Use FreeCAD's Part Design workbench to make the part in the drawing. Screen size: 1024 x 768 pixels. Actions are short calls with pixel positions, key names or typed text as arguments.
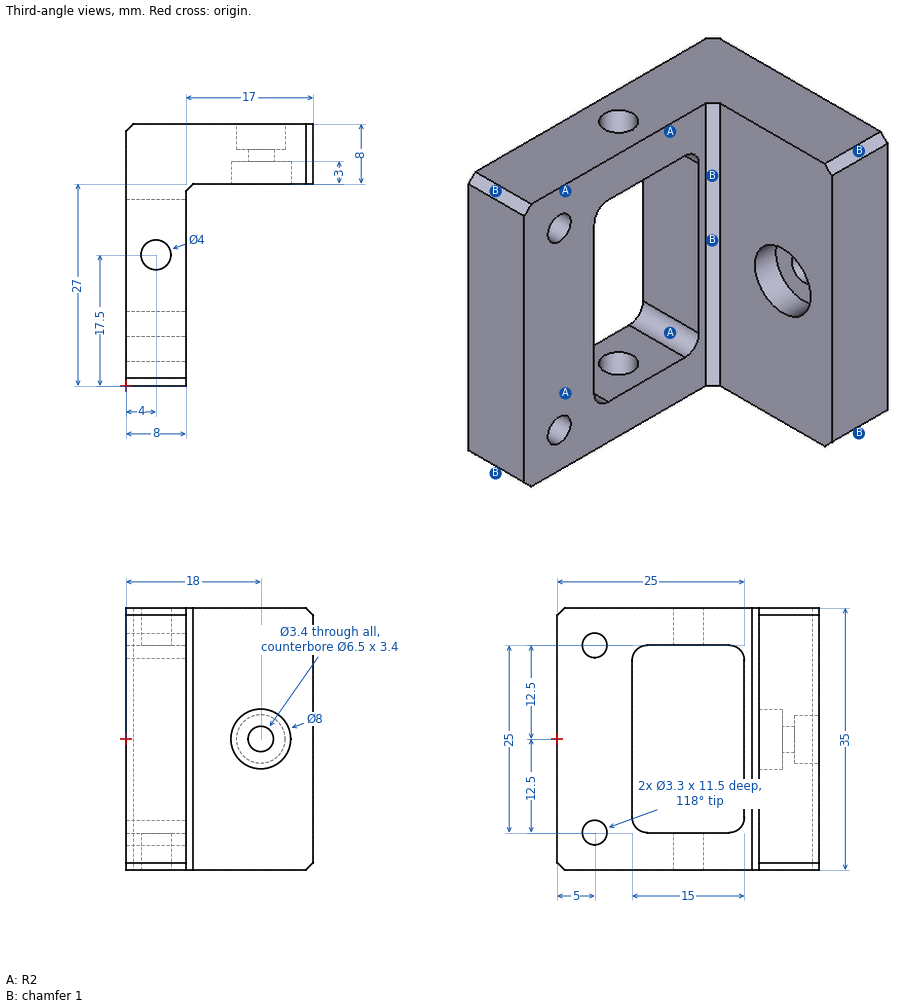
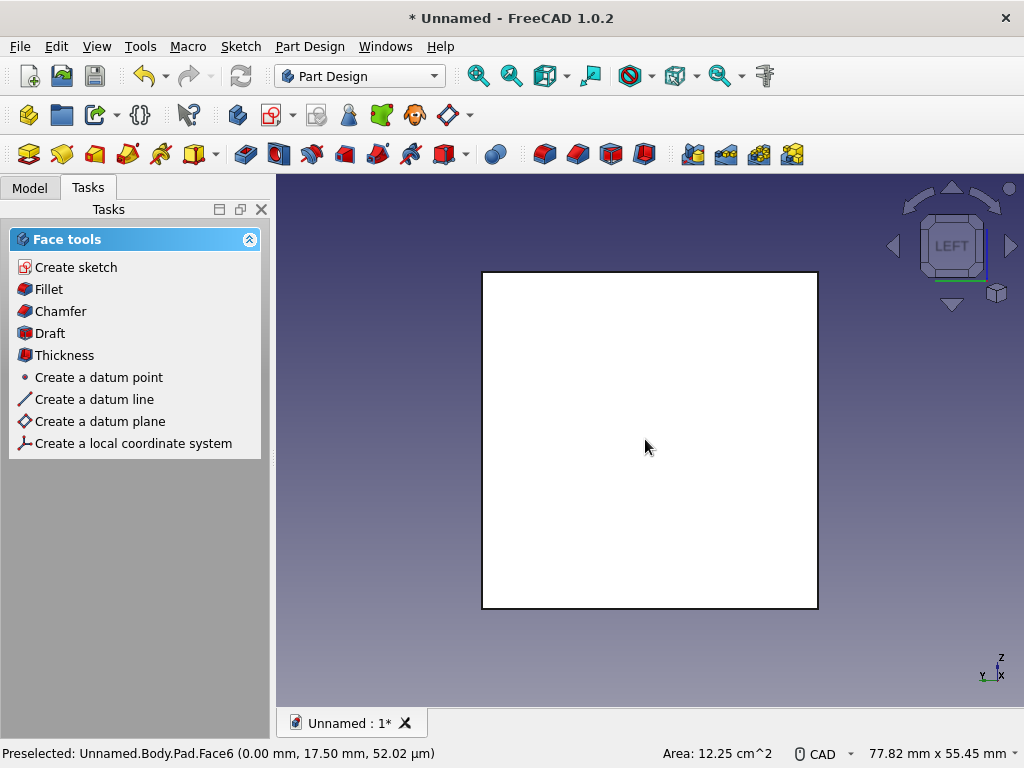
click(270, 116)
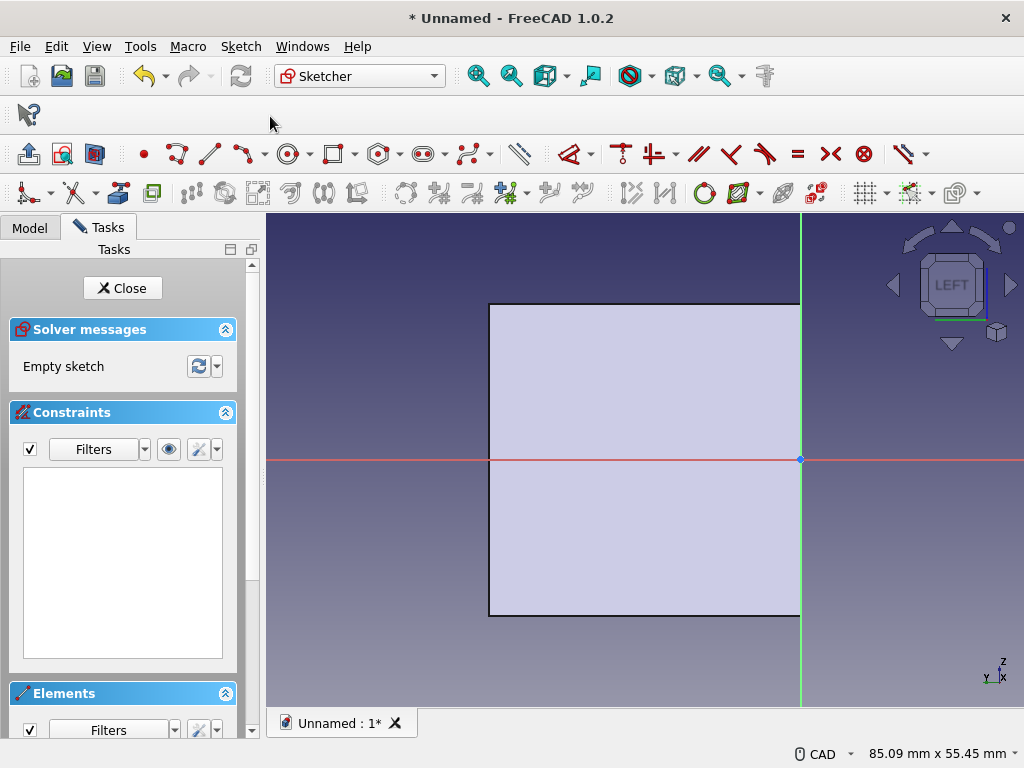
scroll(859, 460, up, 2)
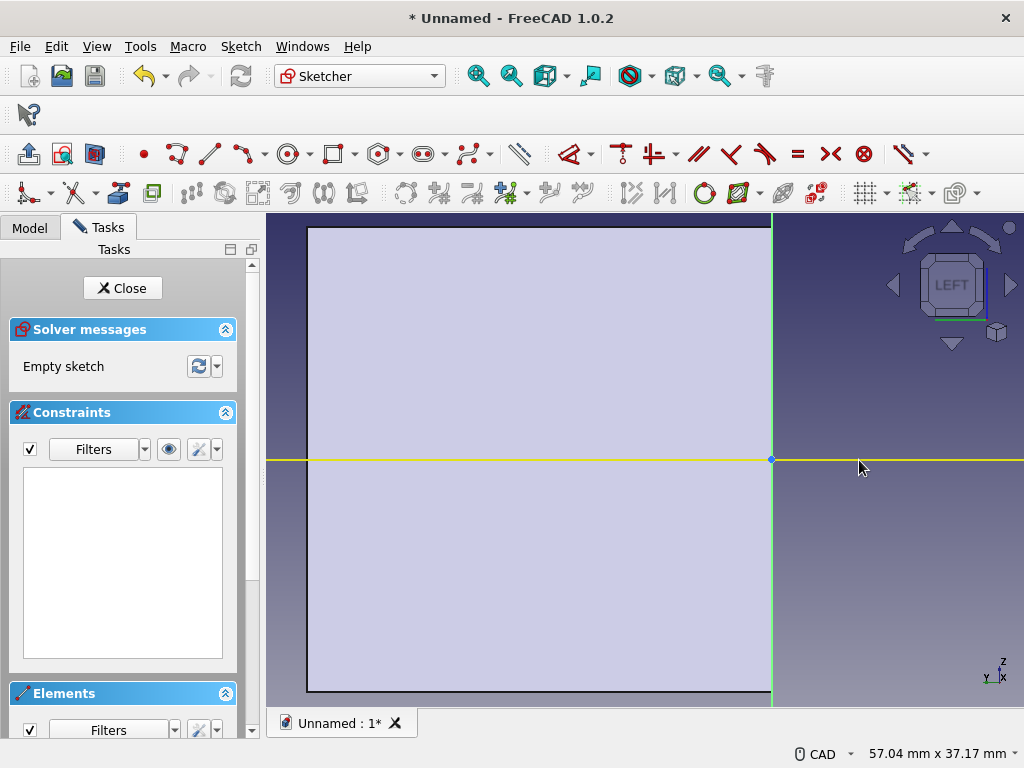
key(g)
key(r)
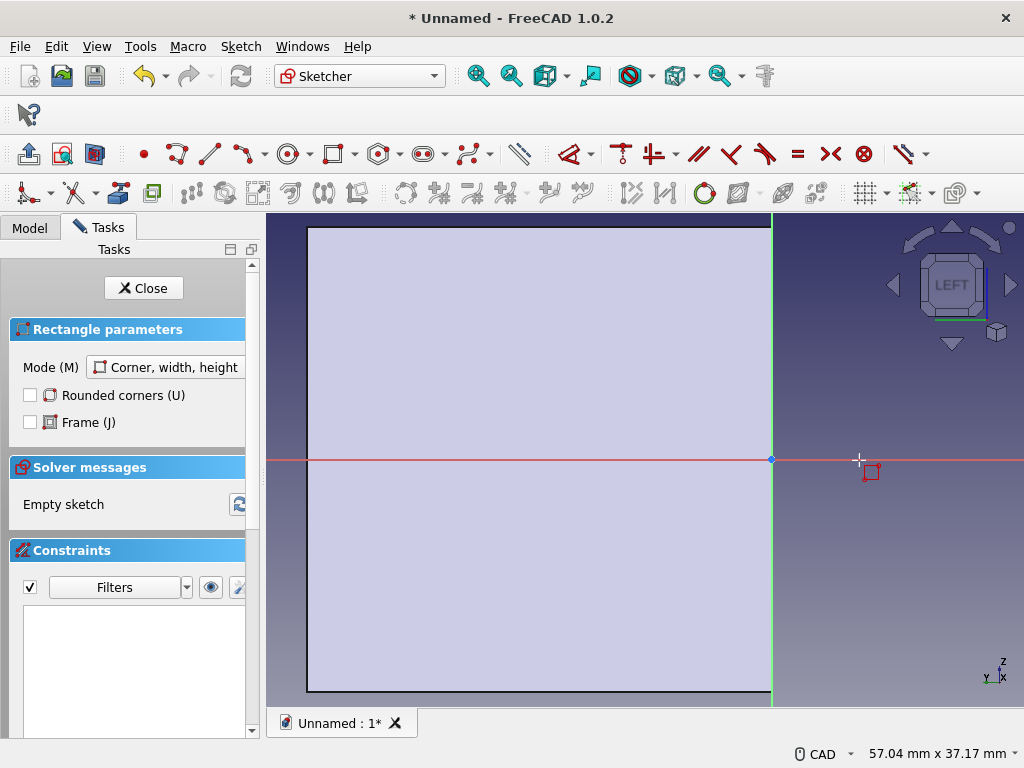
click(440, 294)
move(639, 626)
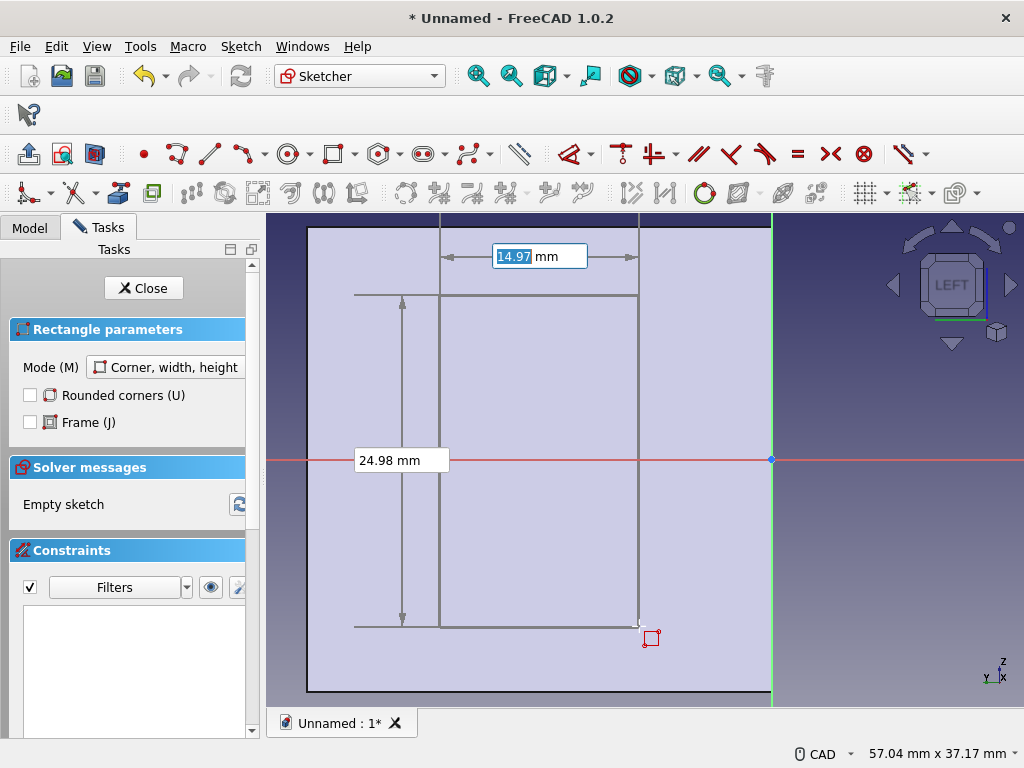
text(15)
key(Tab)
text(25)
key(Return)
key(Escape)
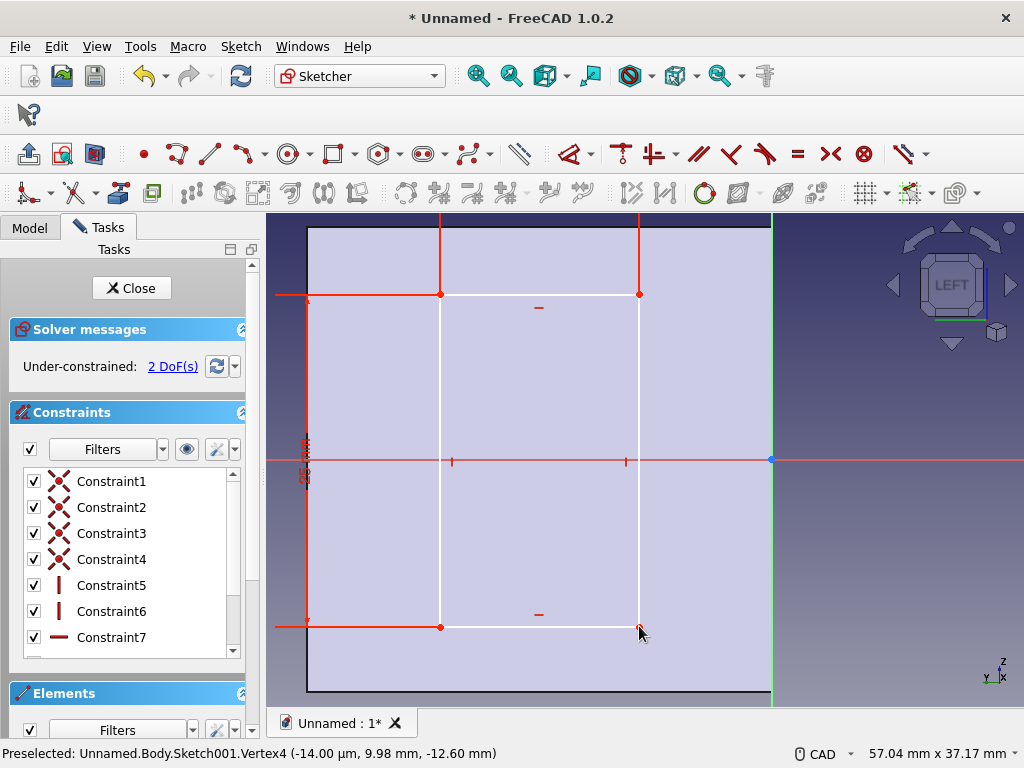
key(d)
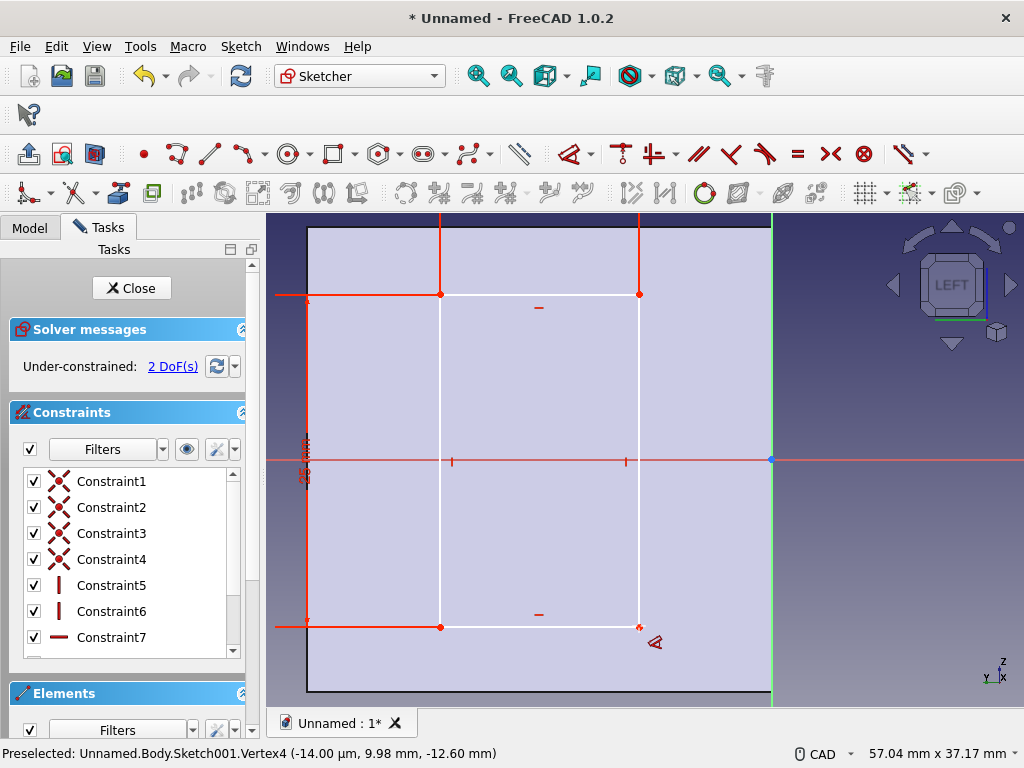
click(440, 295)
click(606, 261)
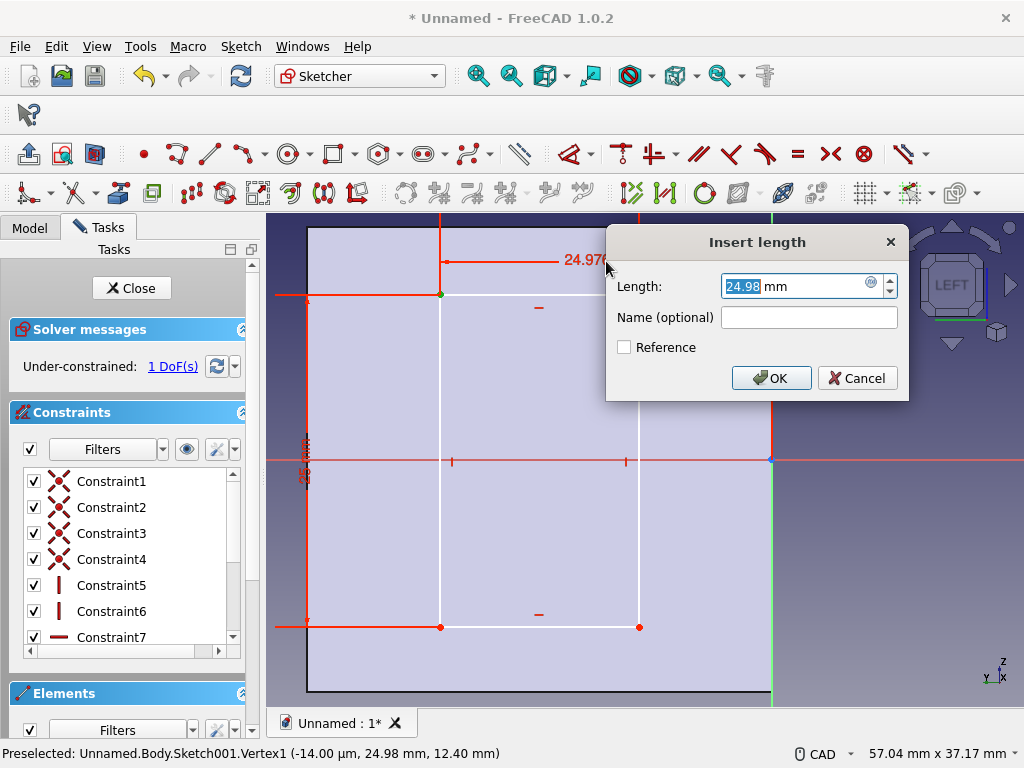
text(25)
key(Return)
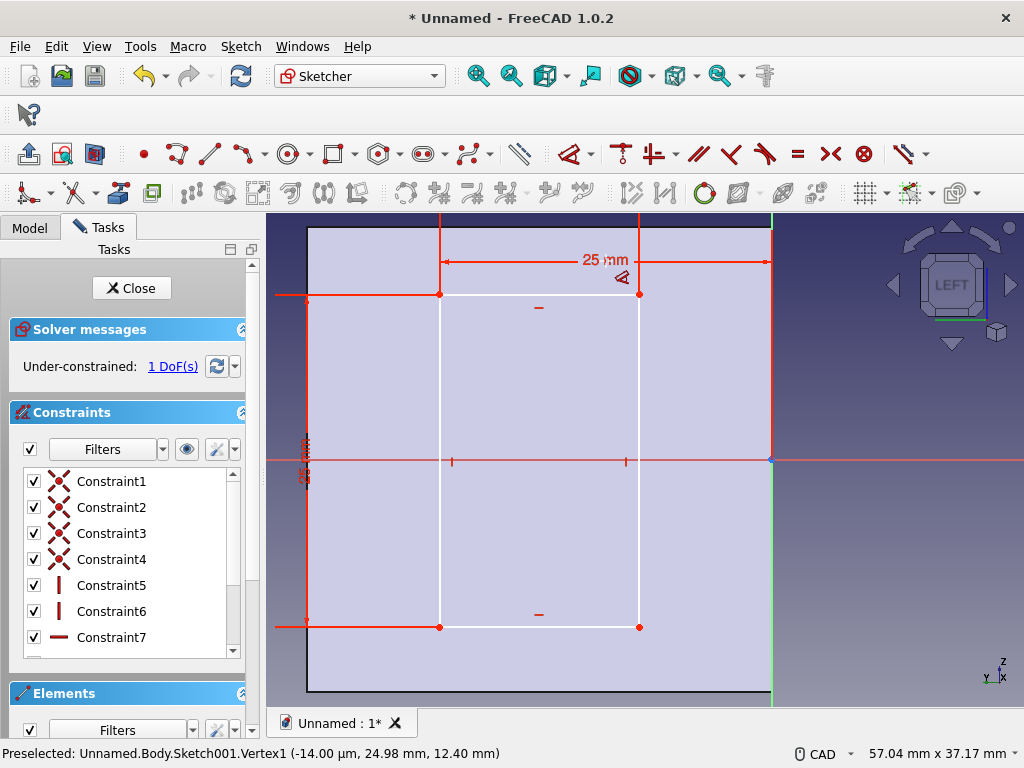
click(440, 295)
click(806, 377)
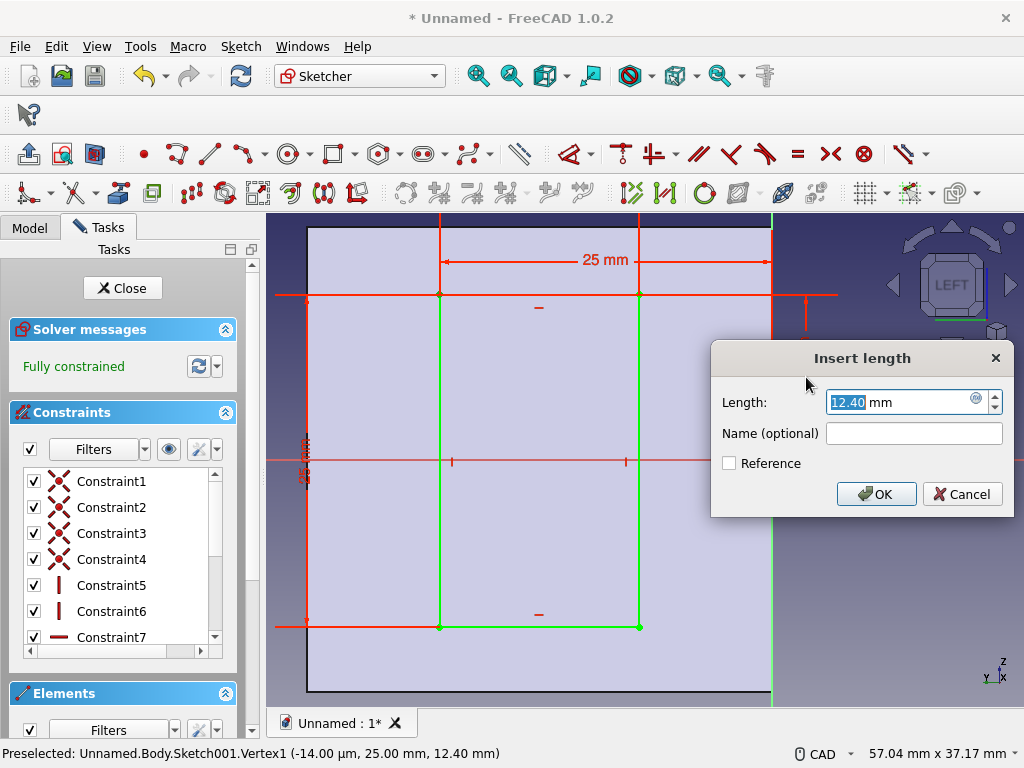
text(12.5)
key(Return)
key(Escape)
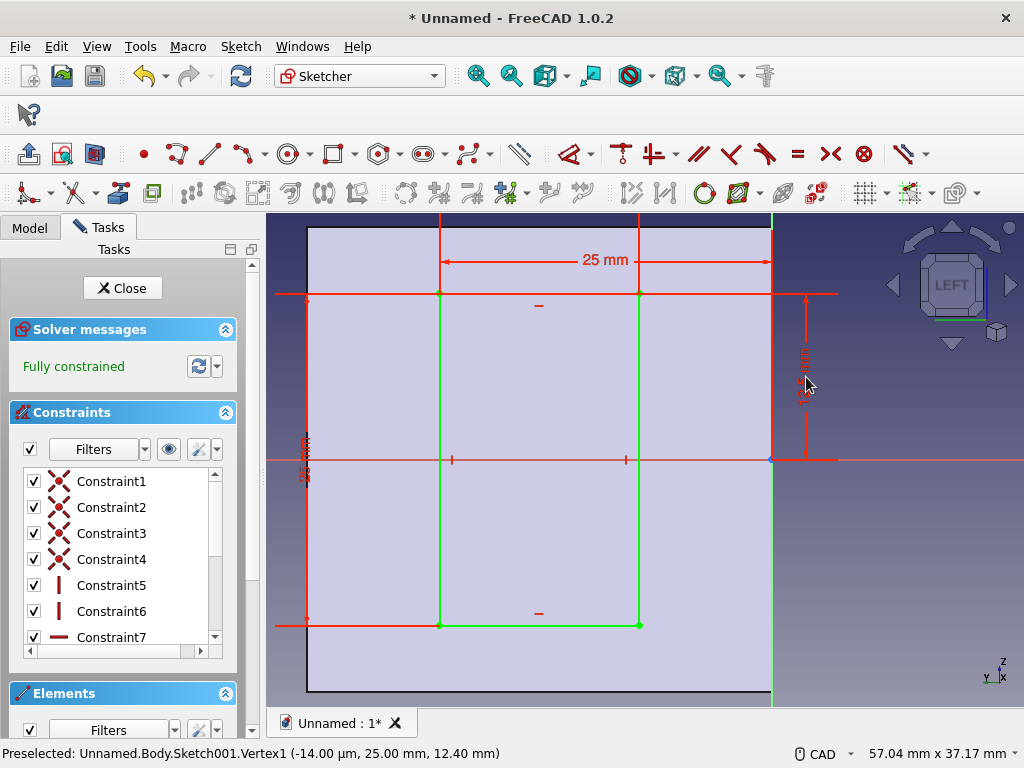
click(123, 288)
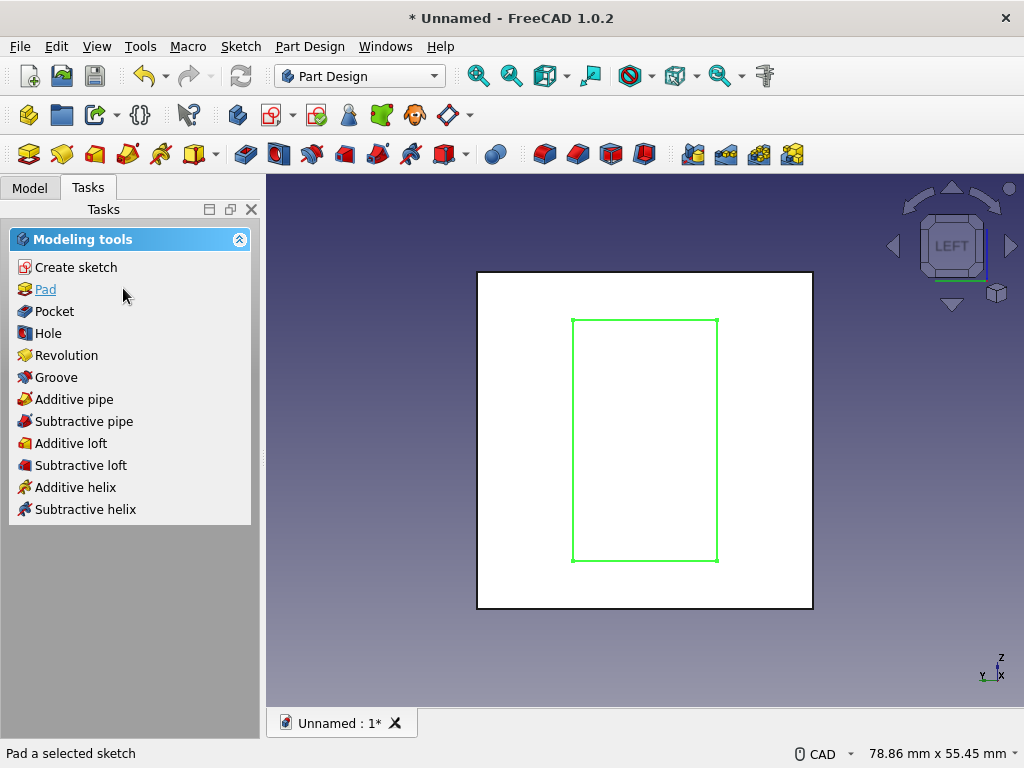
click(246, 154)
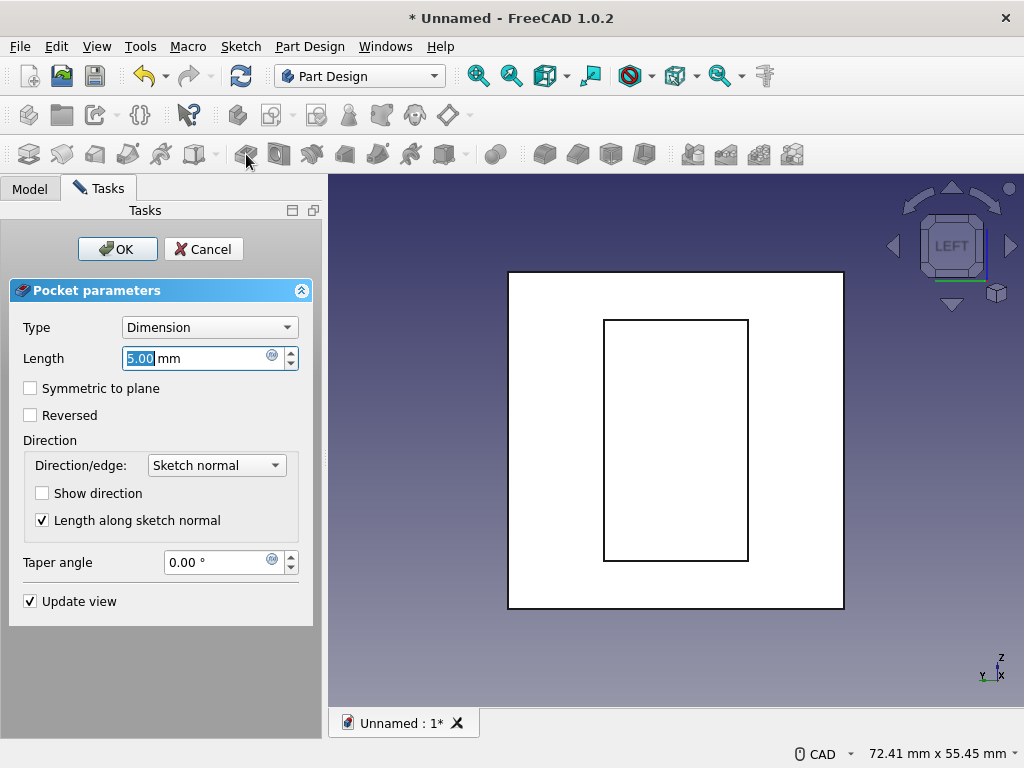
click(210, 328)